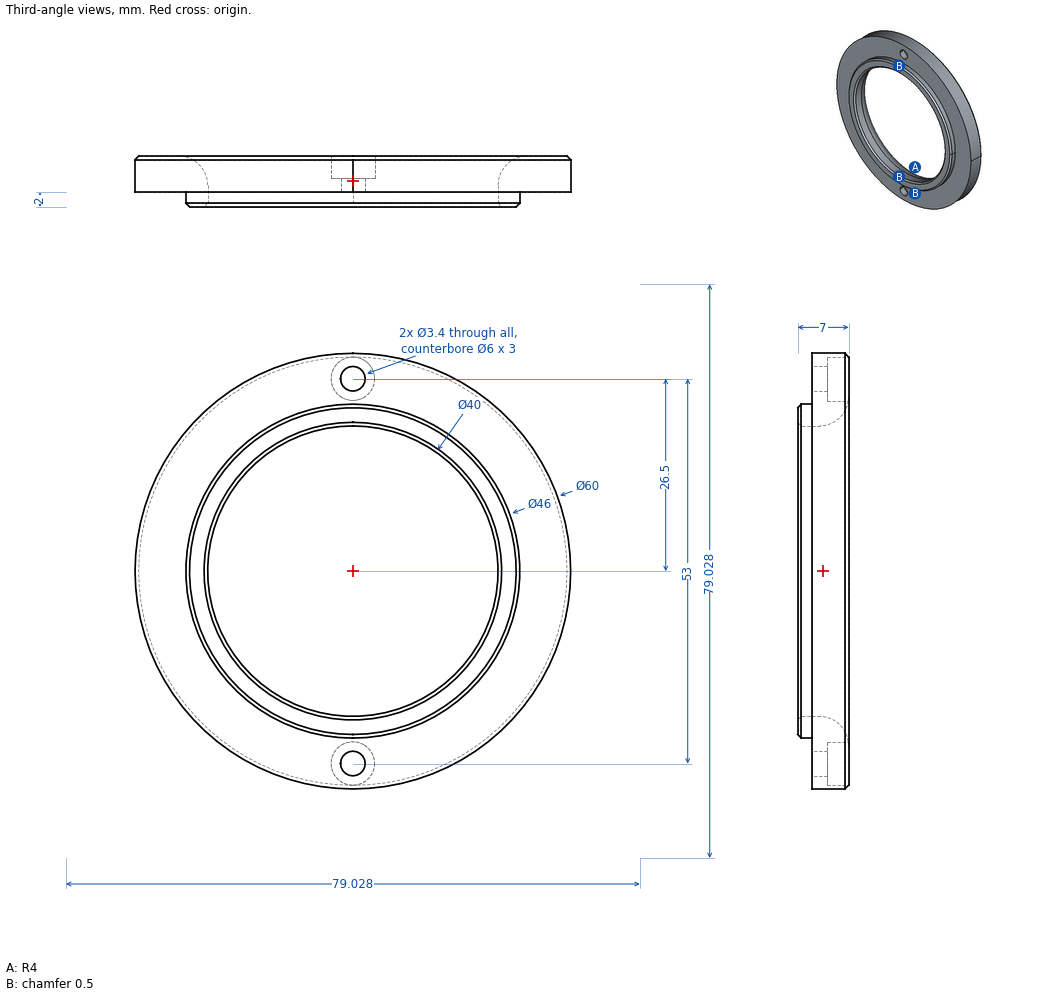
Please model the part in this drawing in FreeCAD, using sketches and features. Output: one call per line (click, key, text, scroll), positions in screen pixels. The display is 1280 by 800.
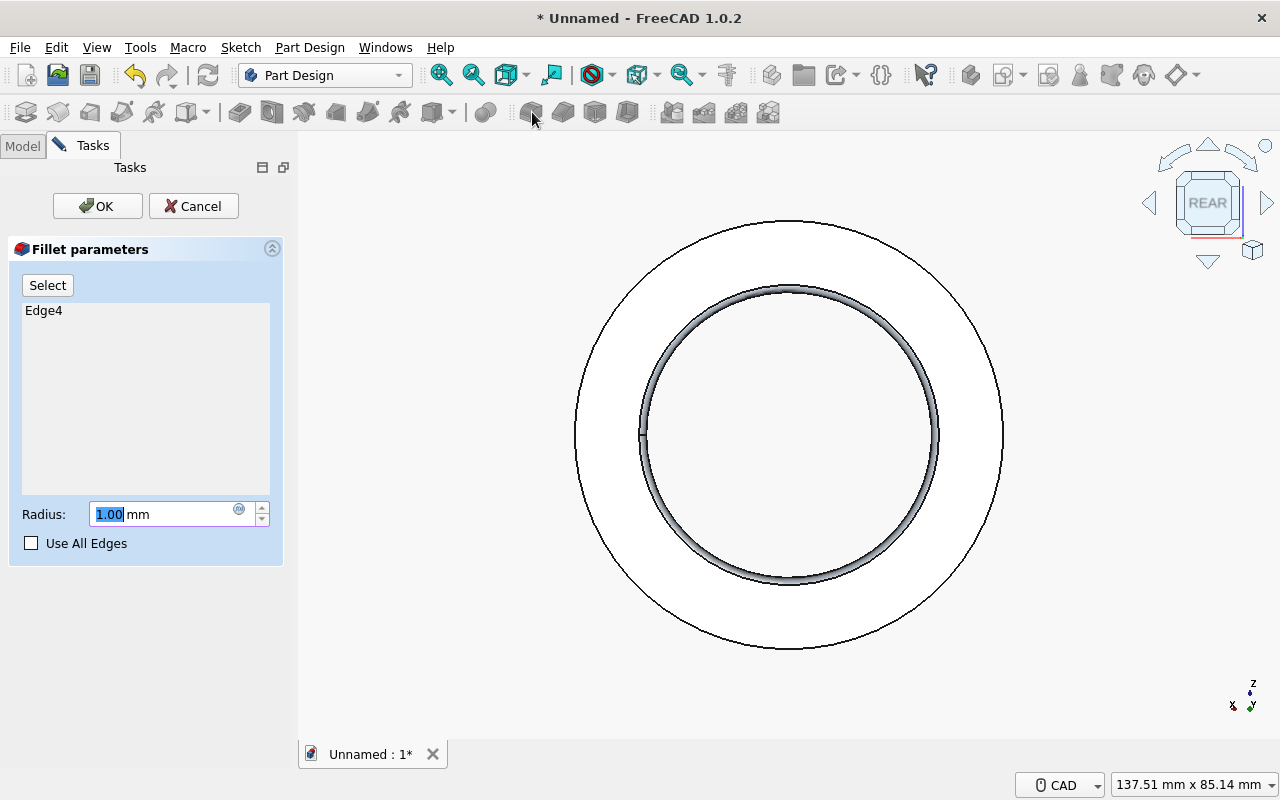
text(4)
key(Tab)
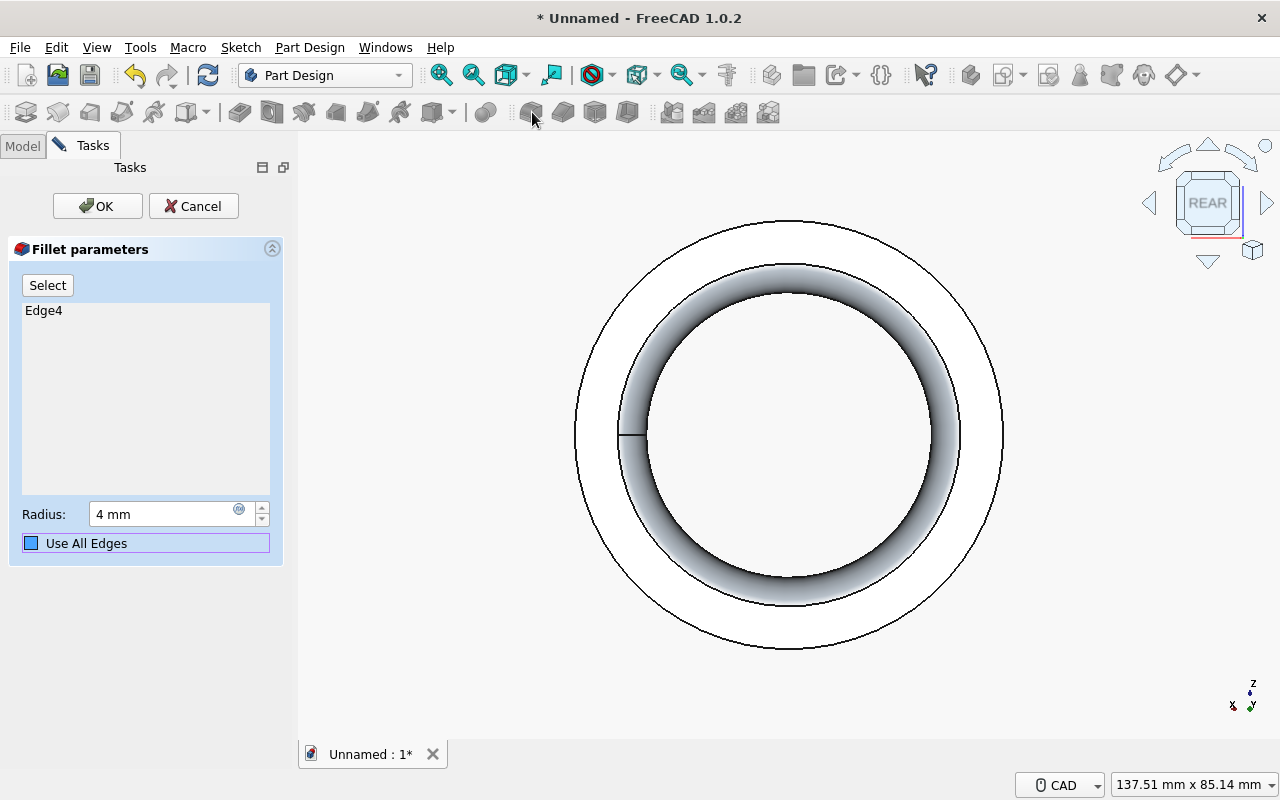
click(98, 206)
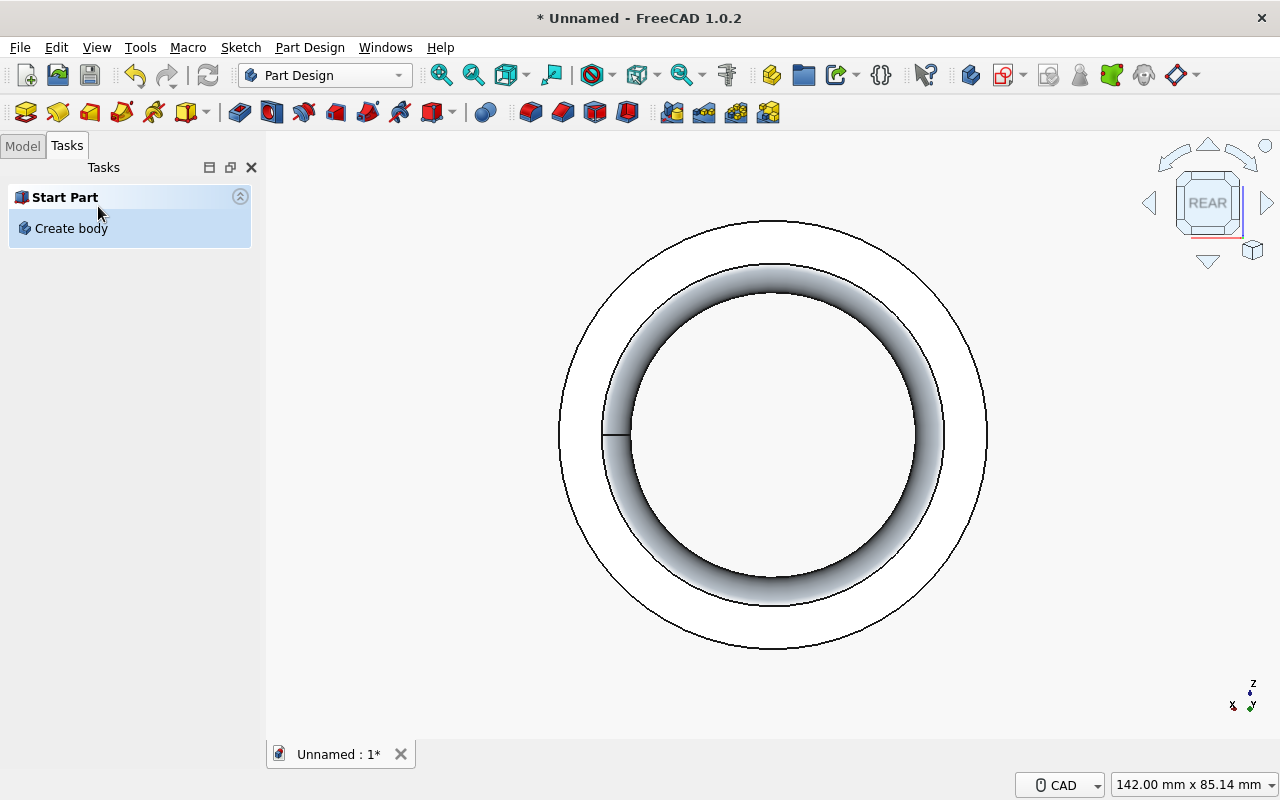
click(987, 434)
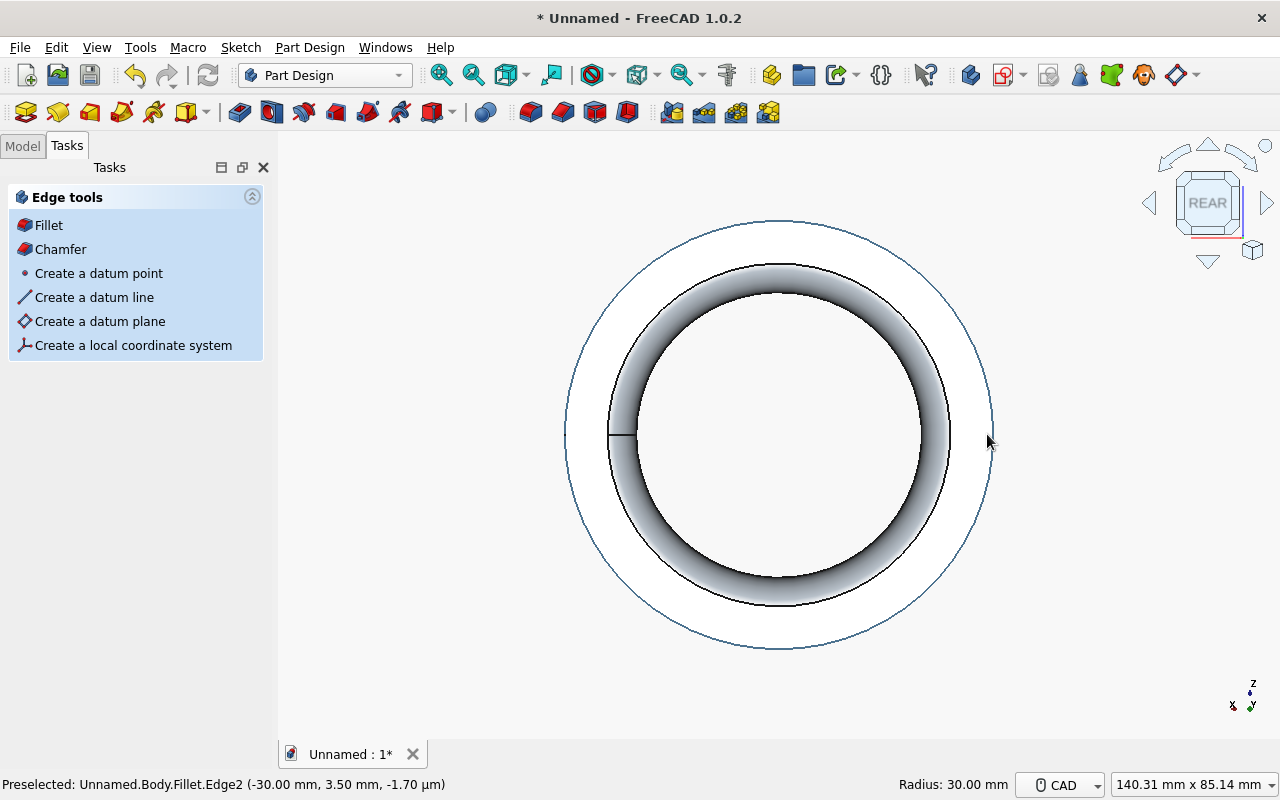
key(0)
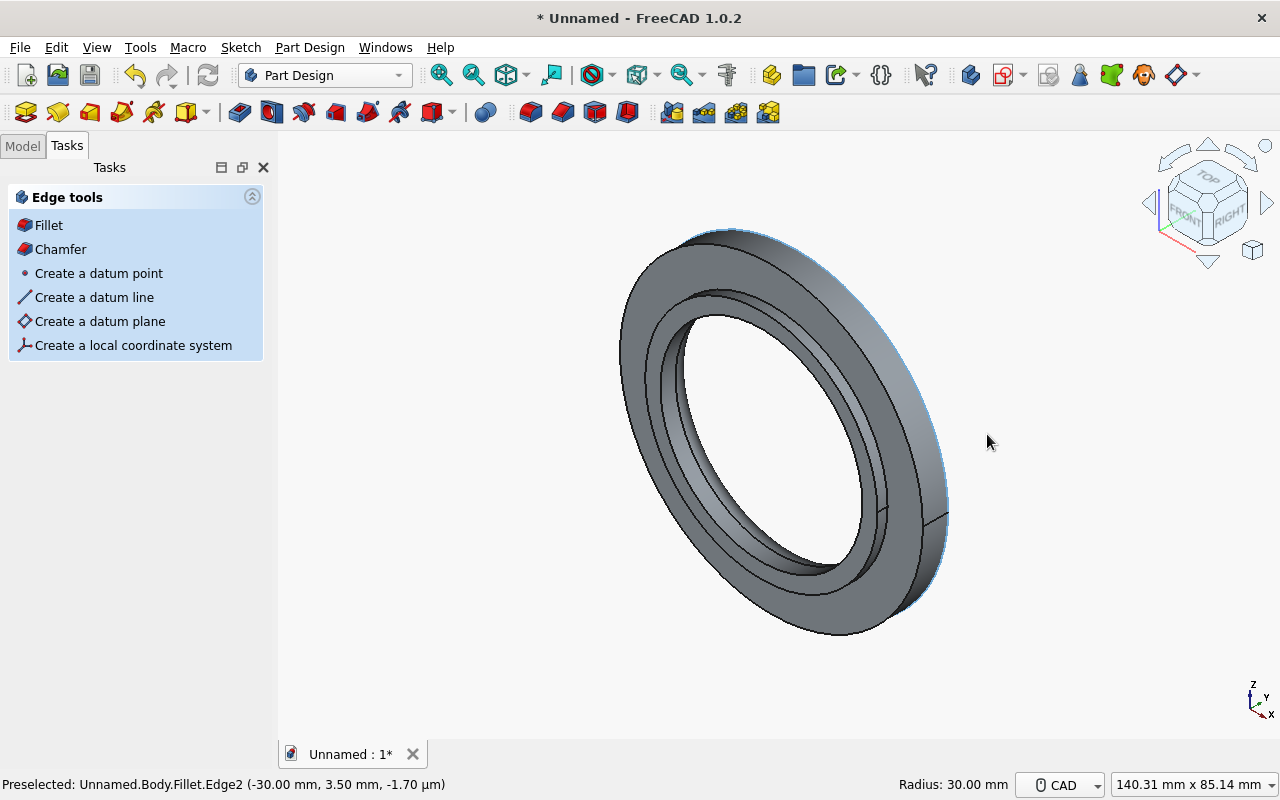
click(725, 296, ctrl)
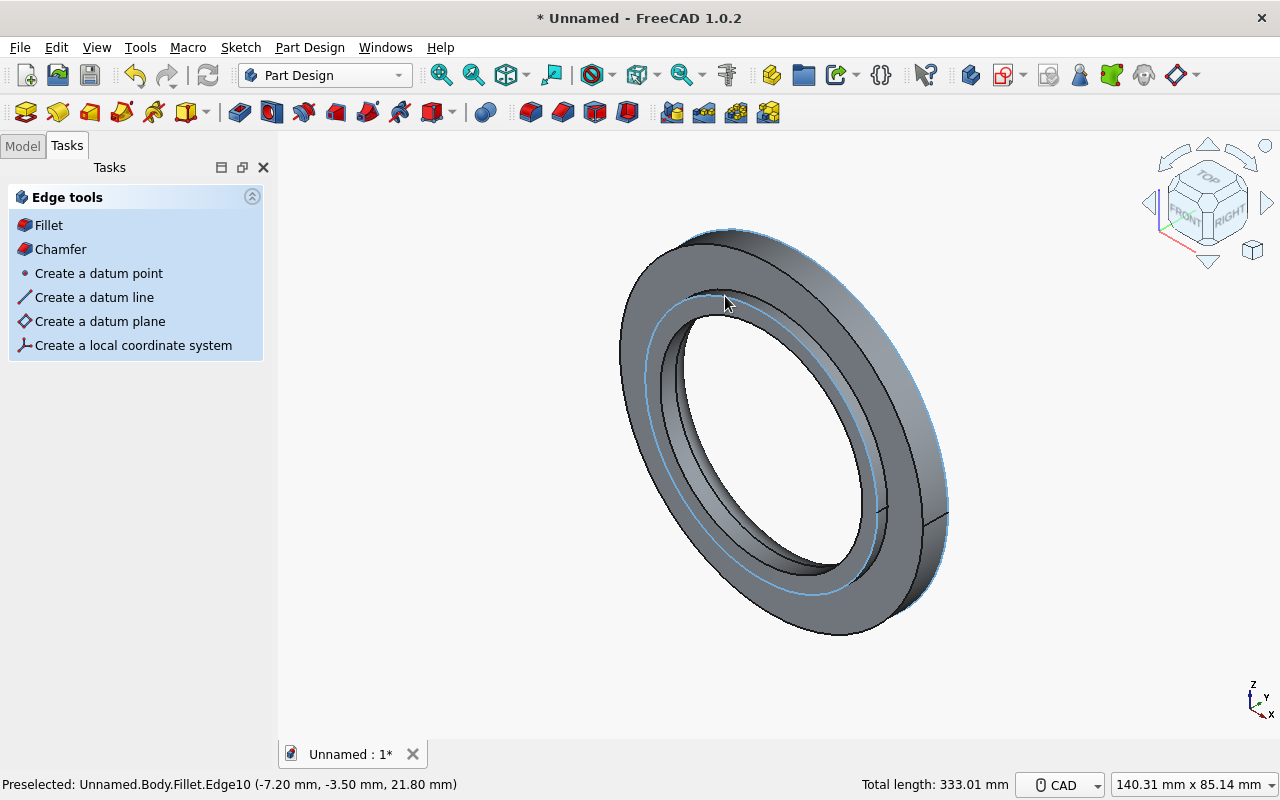
click(660, 386, ctrl)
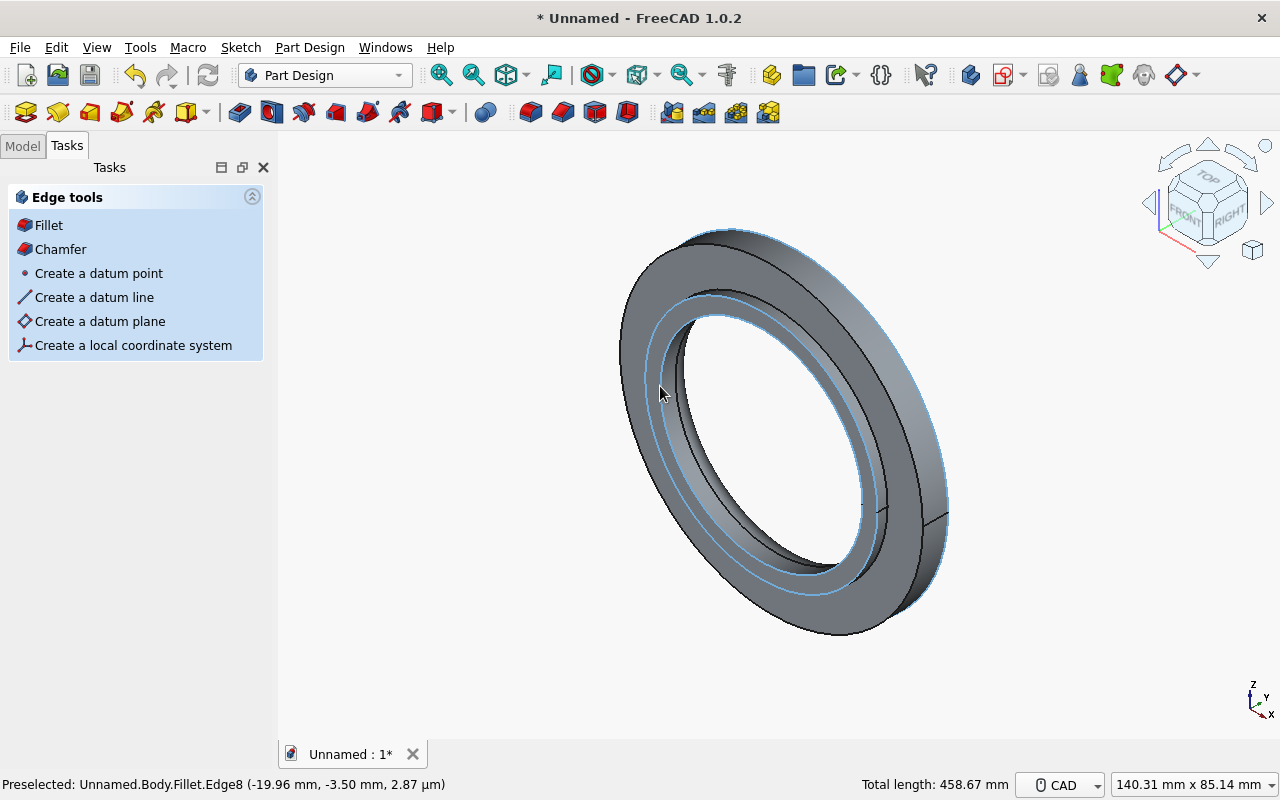
click(564, 112)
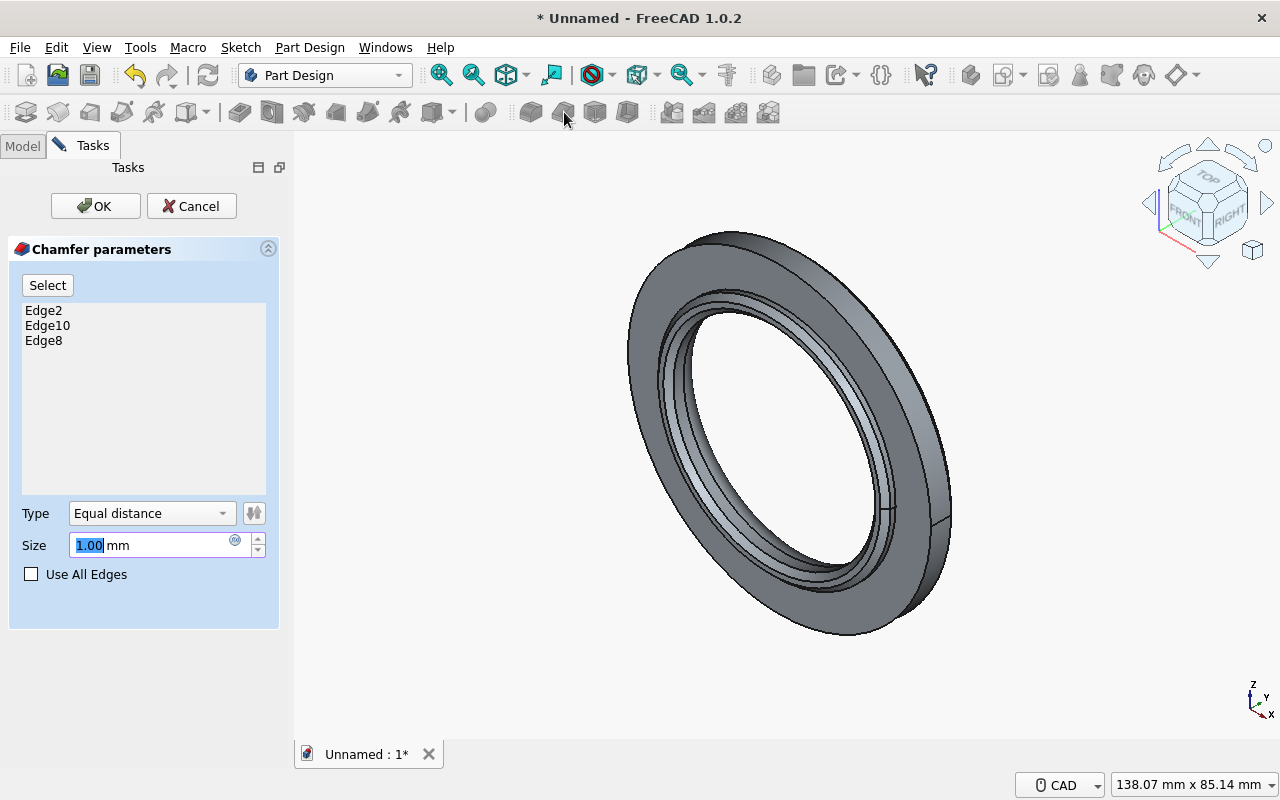
text(0.5)
key(Tab)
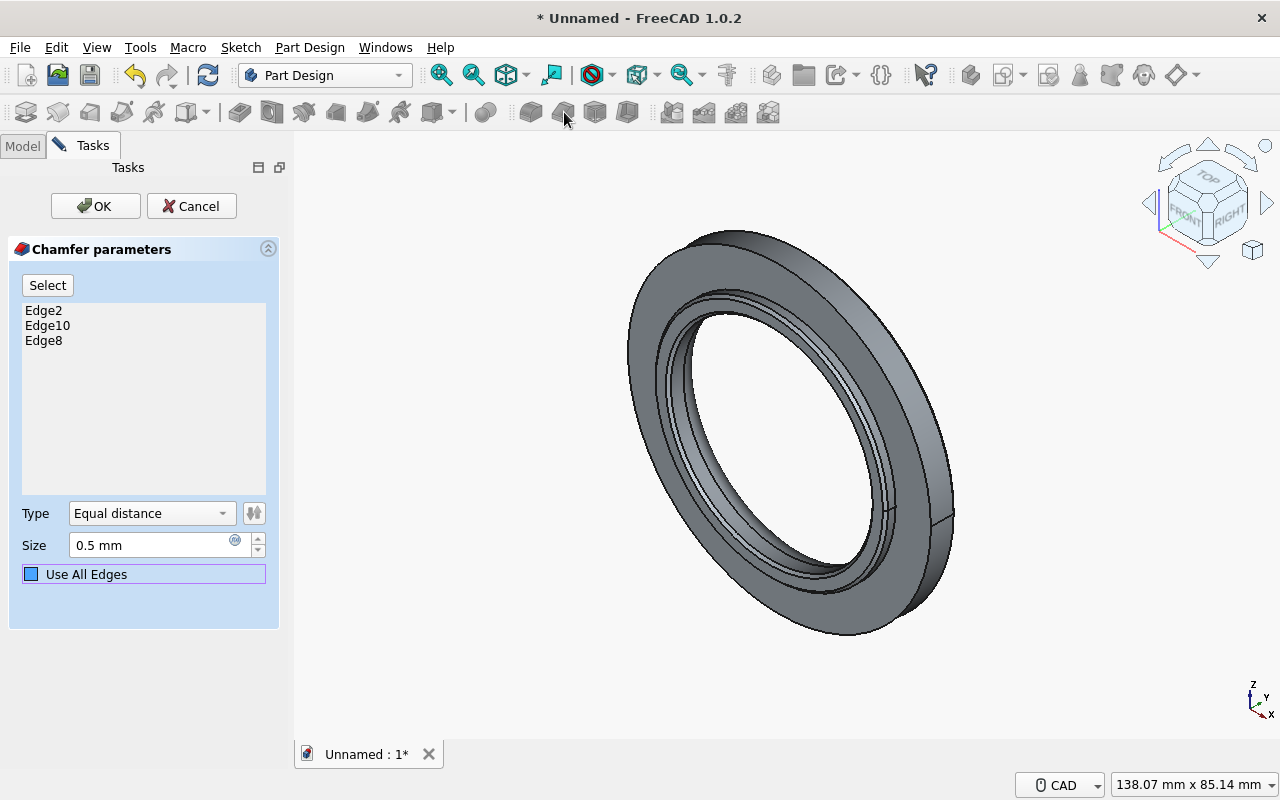
click(96, 206)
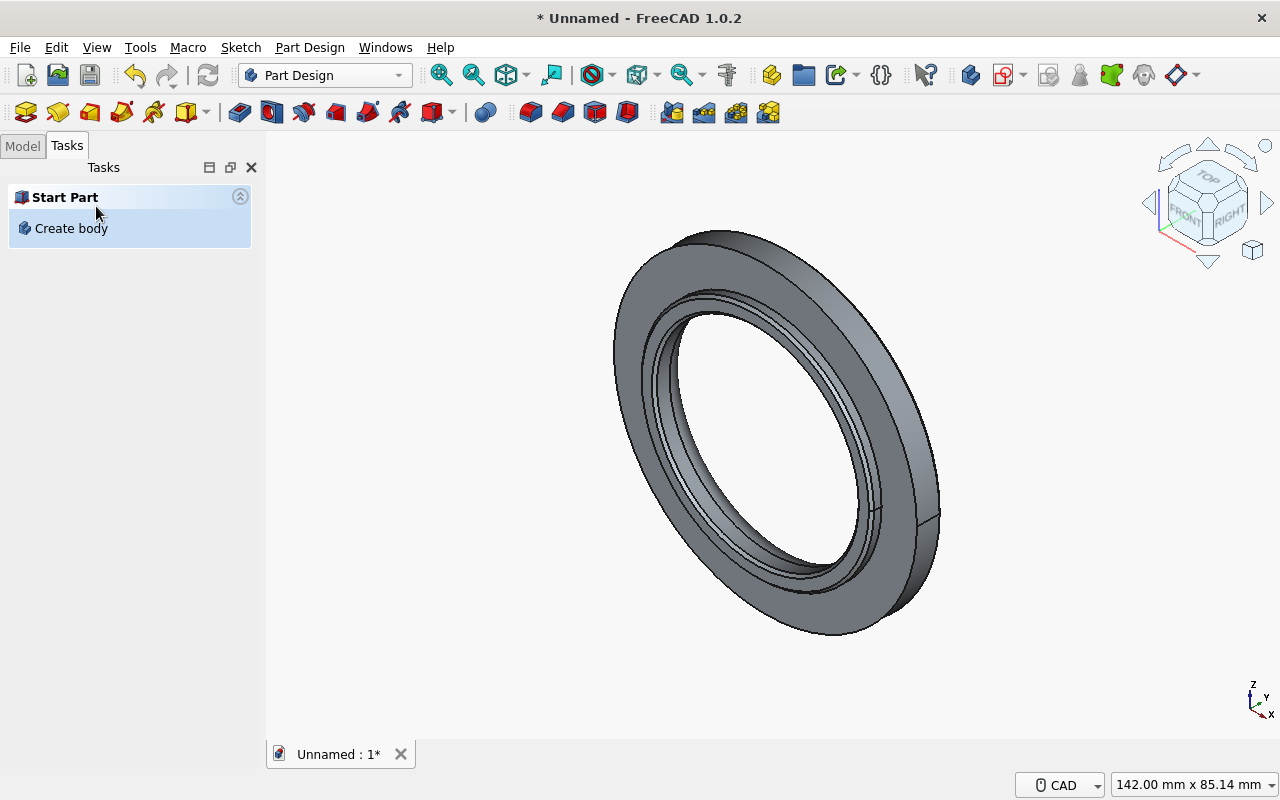
key(4)